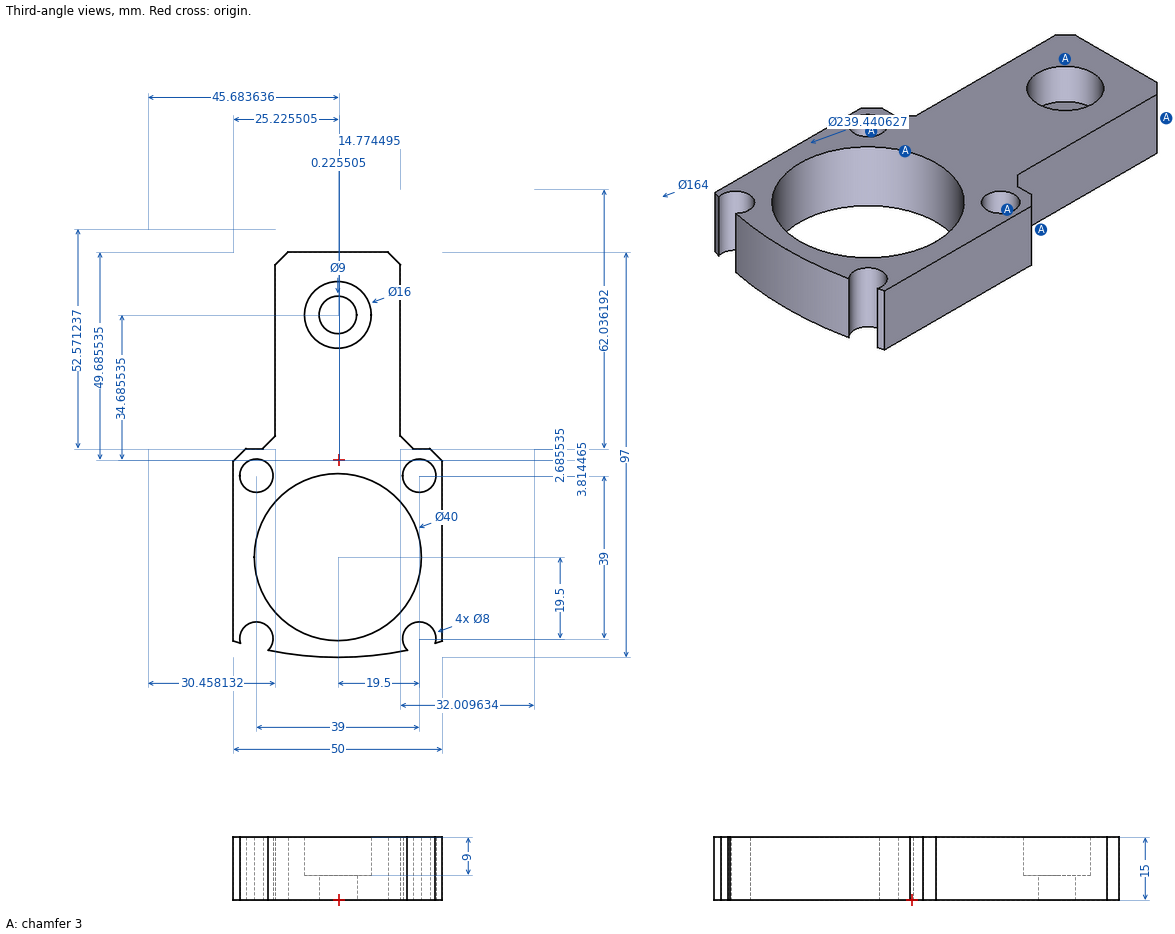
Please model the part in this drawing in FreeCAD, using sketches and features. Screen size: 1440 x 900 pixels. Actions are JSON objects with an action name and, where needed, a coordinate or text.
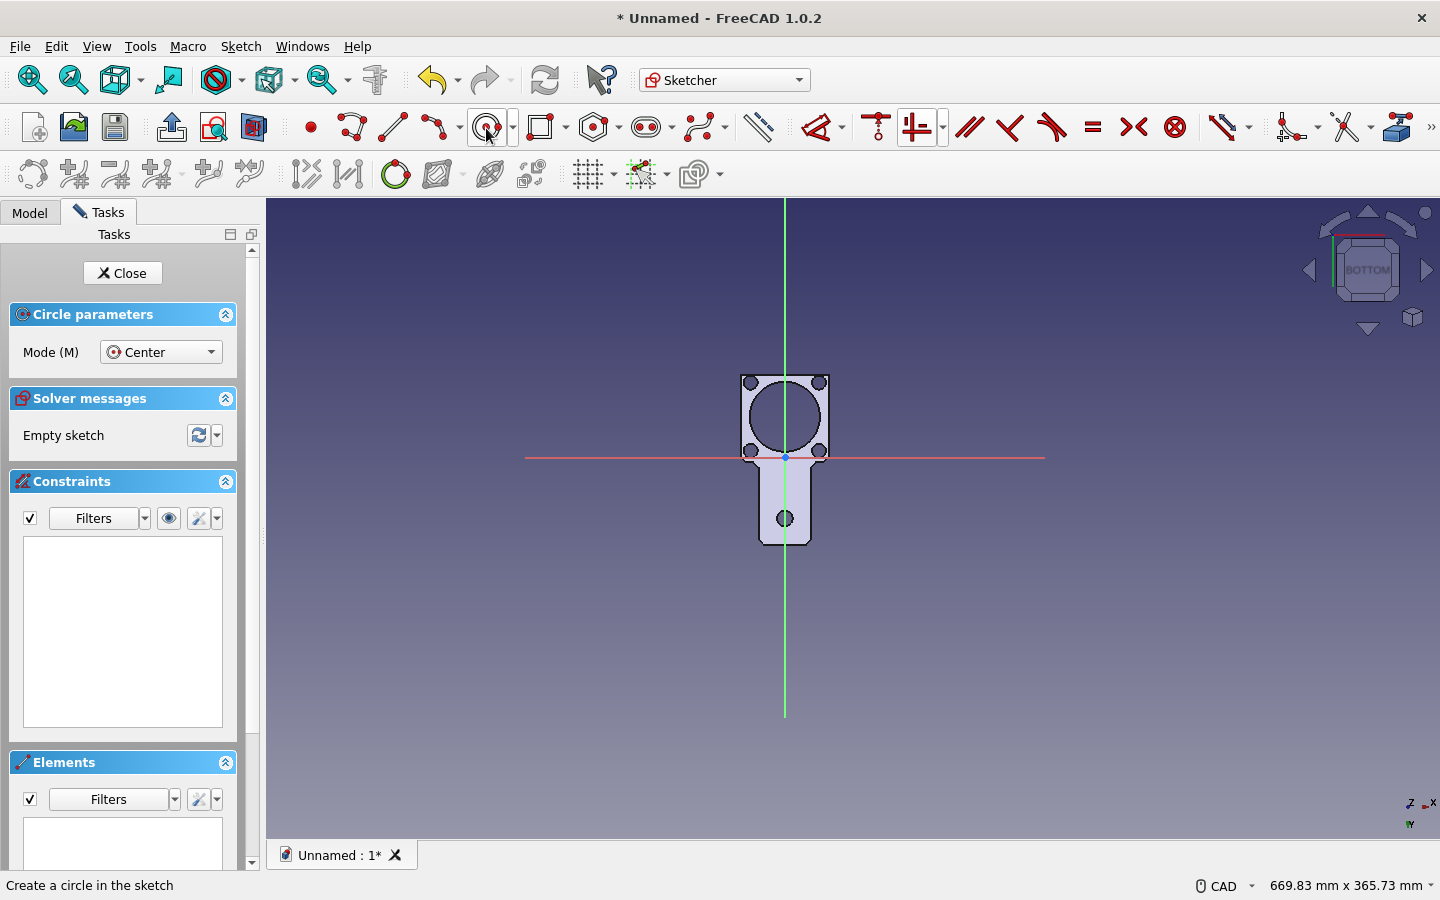
{"action": "scroll", "coordinate": [785, 518], "scroll_direction": "up", "scroll_amount": 19}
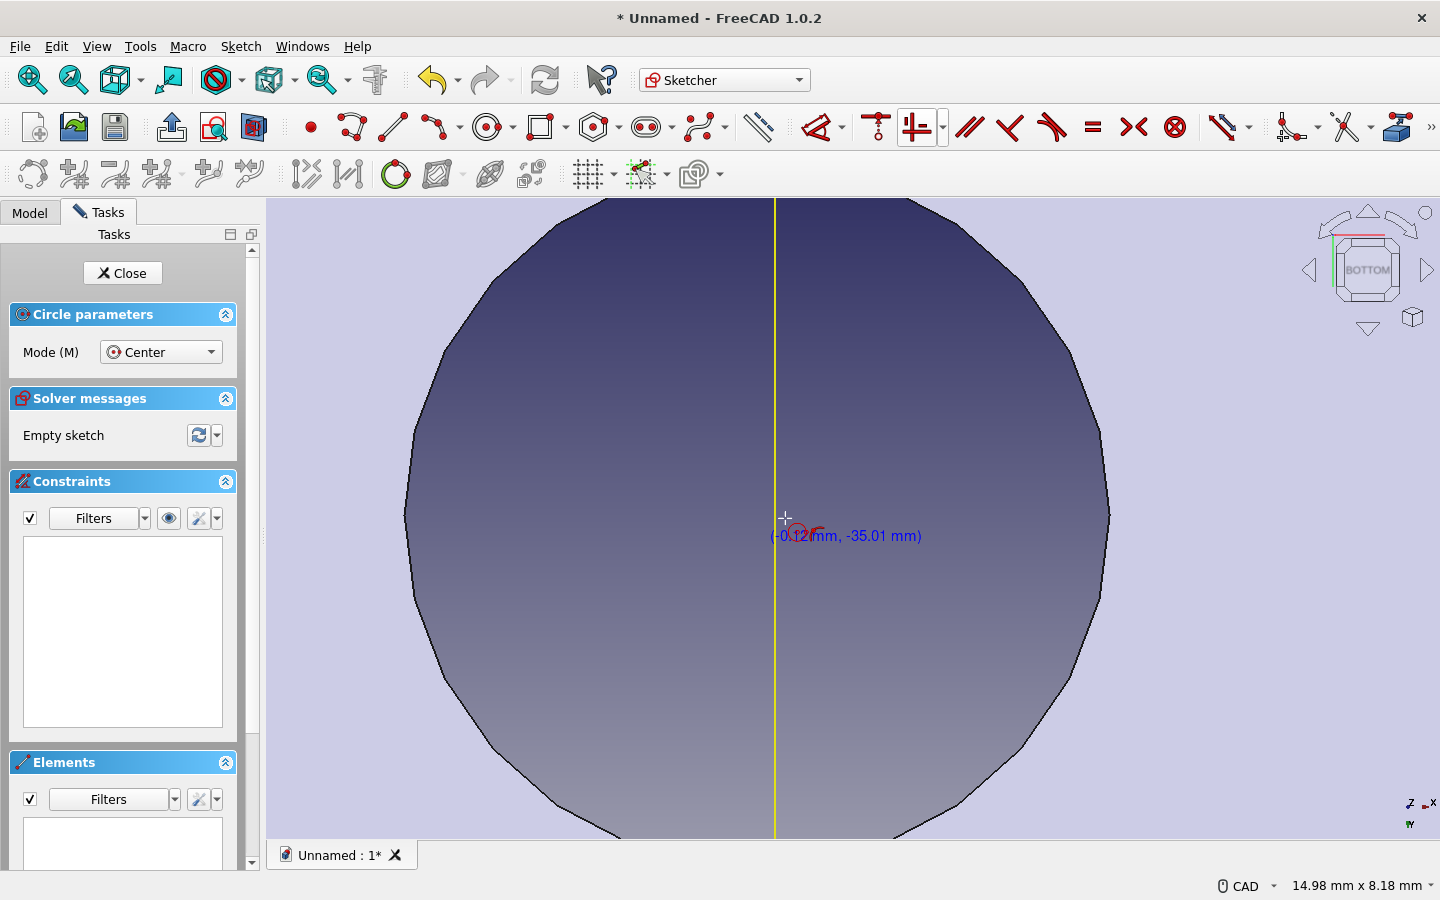
{"action": "left_click", "coordinate": [757, 515]}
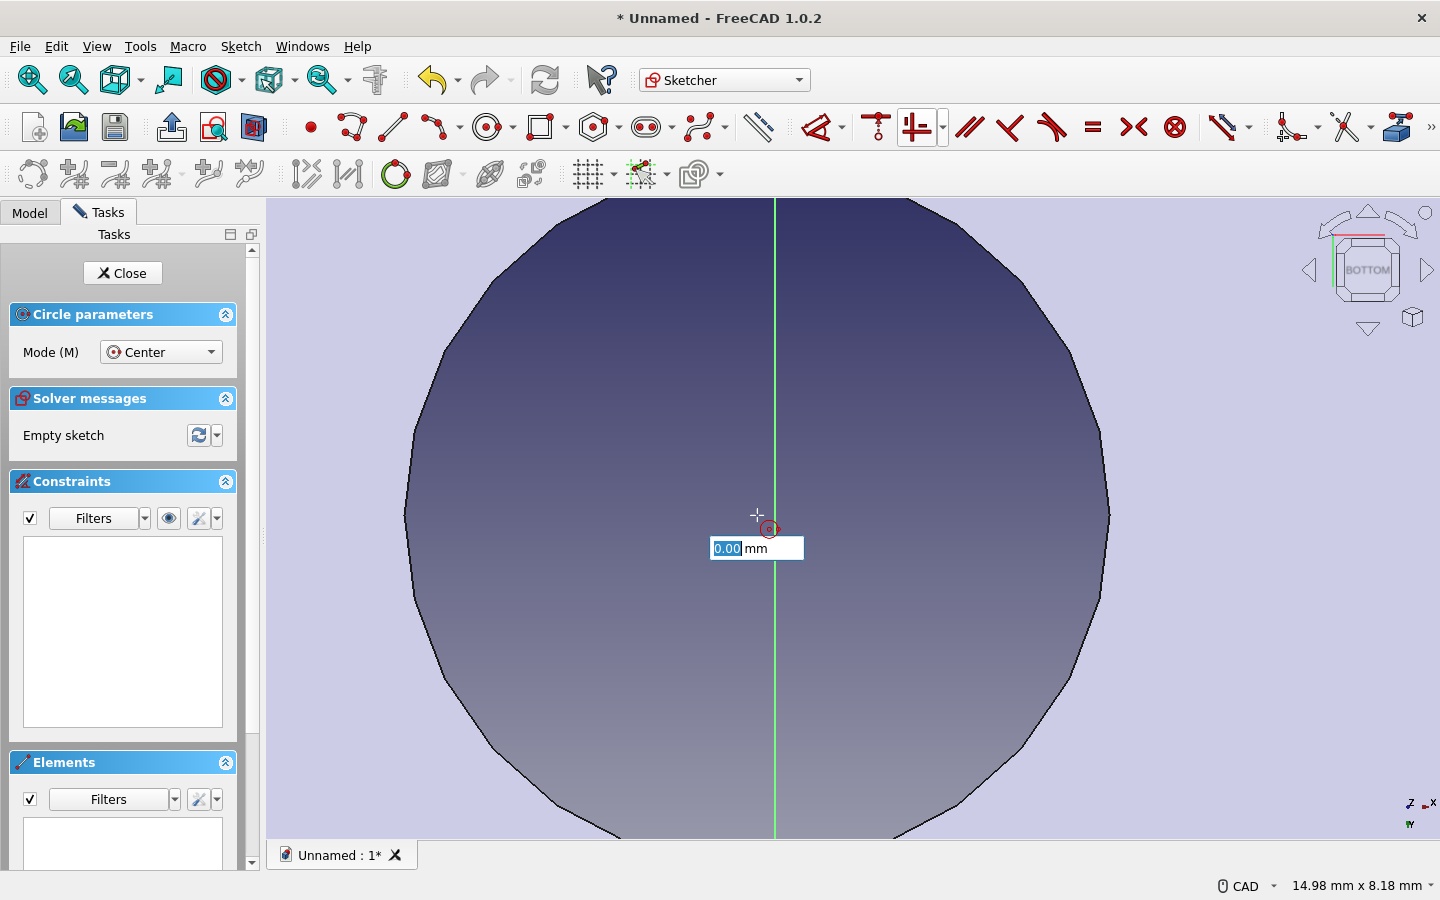
{"action": "scroll", "coordinate": [785, 519], "scroll_direction": "down", "scroll_amount": 18}
{"action": "mouse_move", "coordinate": [966, 338]}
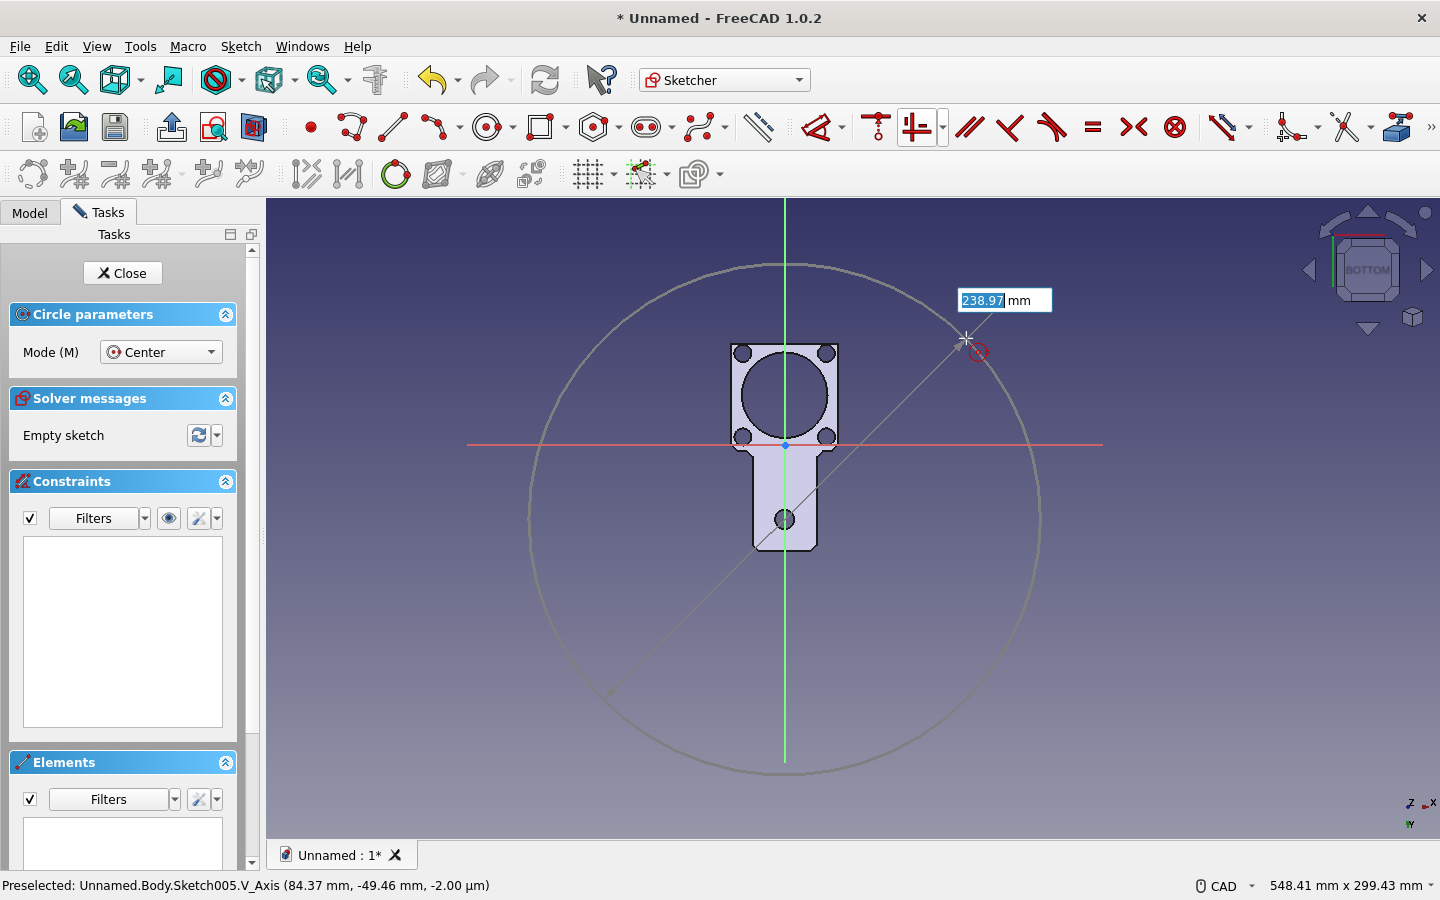
{"action": "type", "text": "239.440627"}
{"action": "key", "text": "Return"}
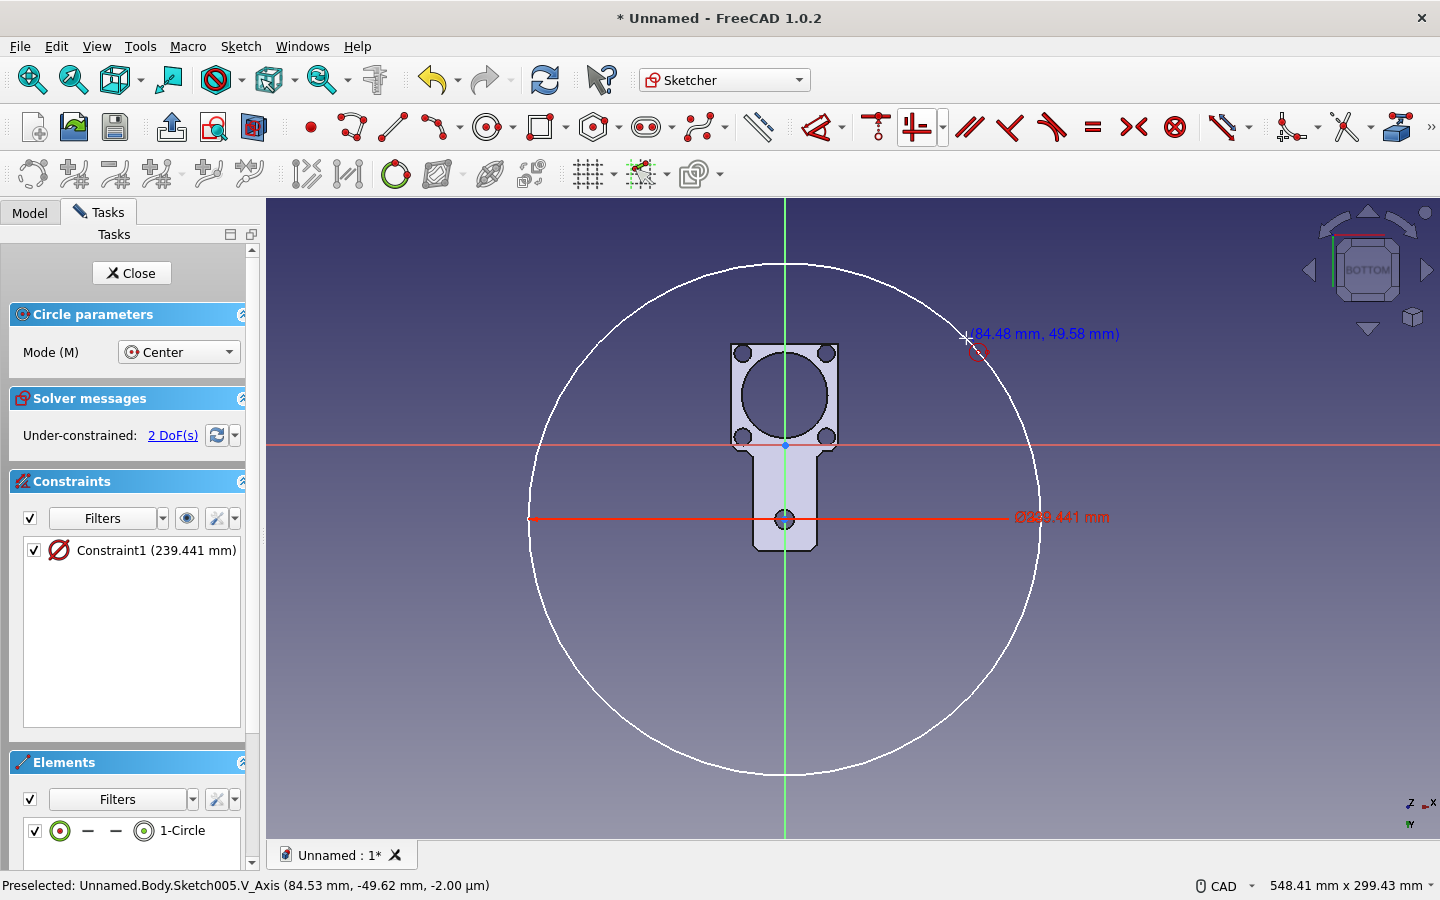
{"action": "scroll", "coordinate": [785, 519], "scroll_direction": "up", "scroll_amount": 18}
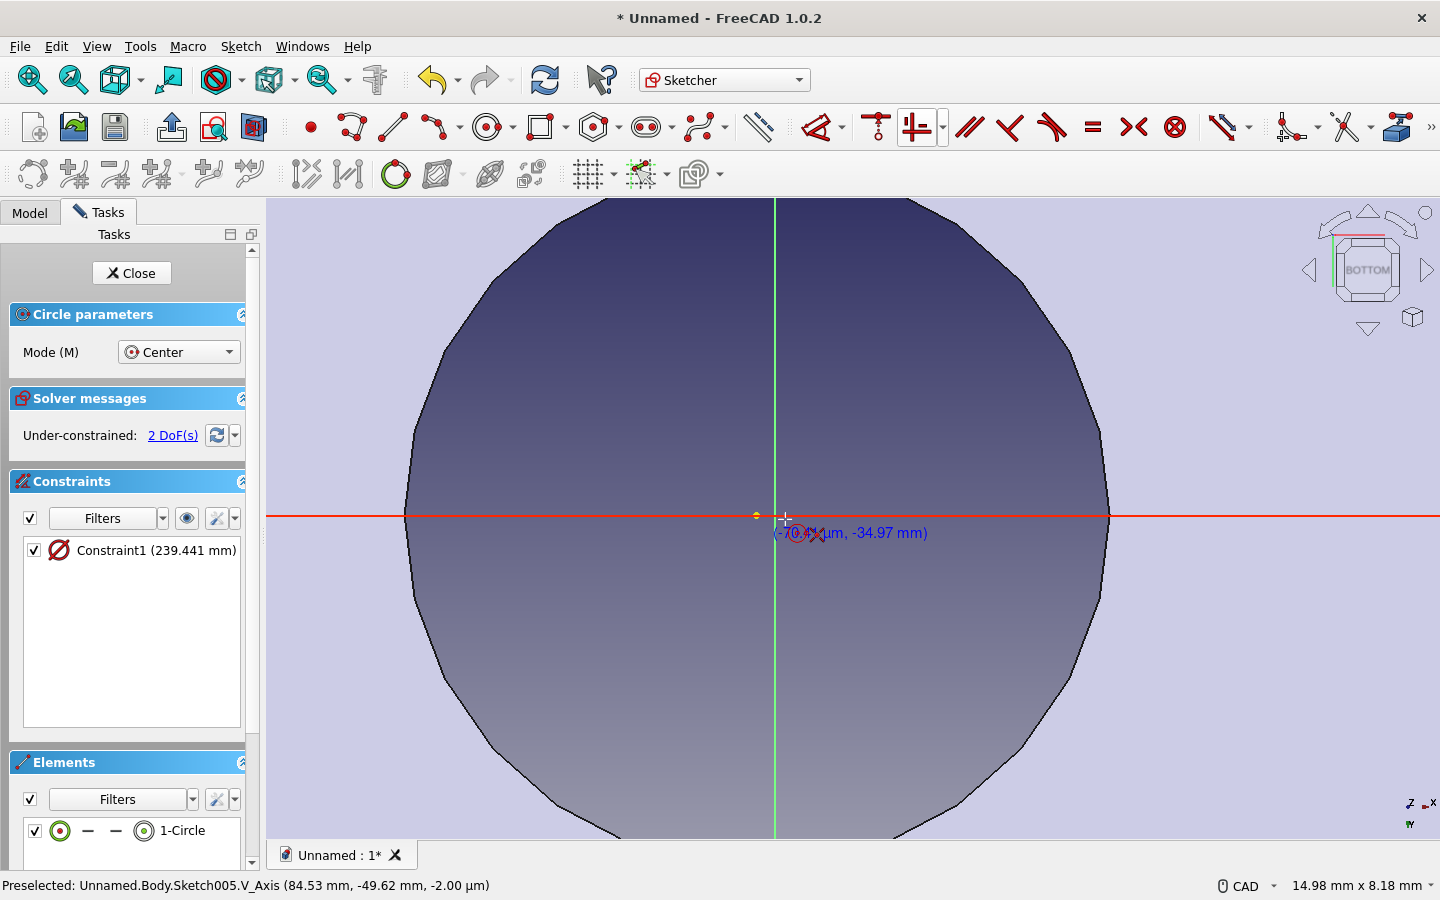
{"action": "left_click", "coordinate": [757, 516]}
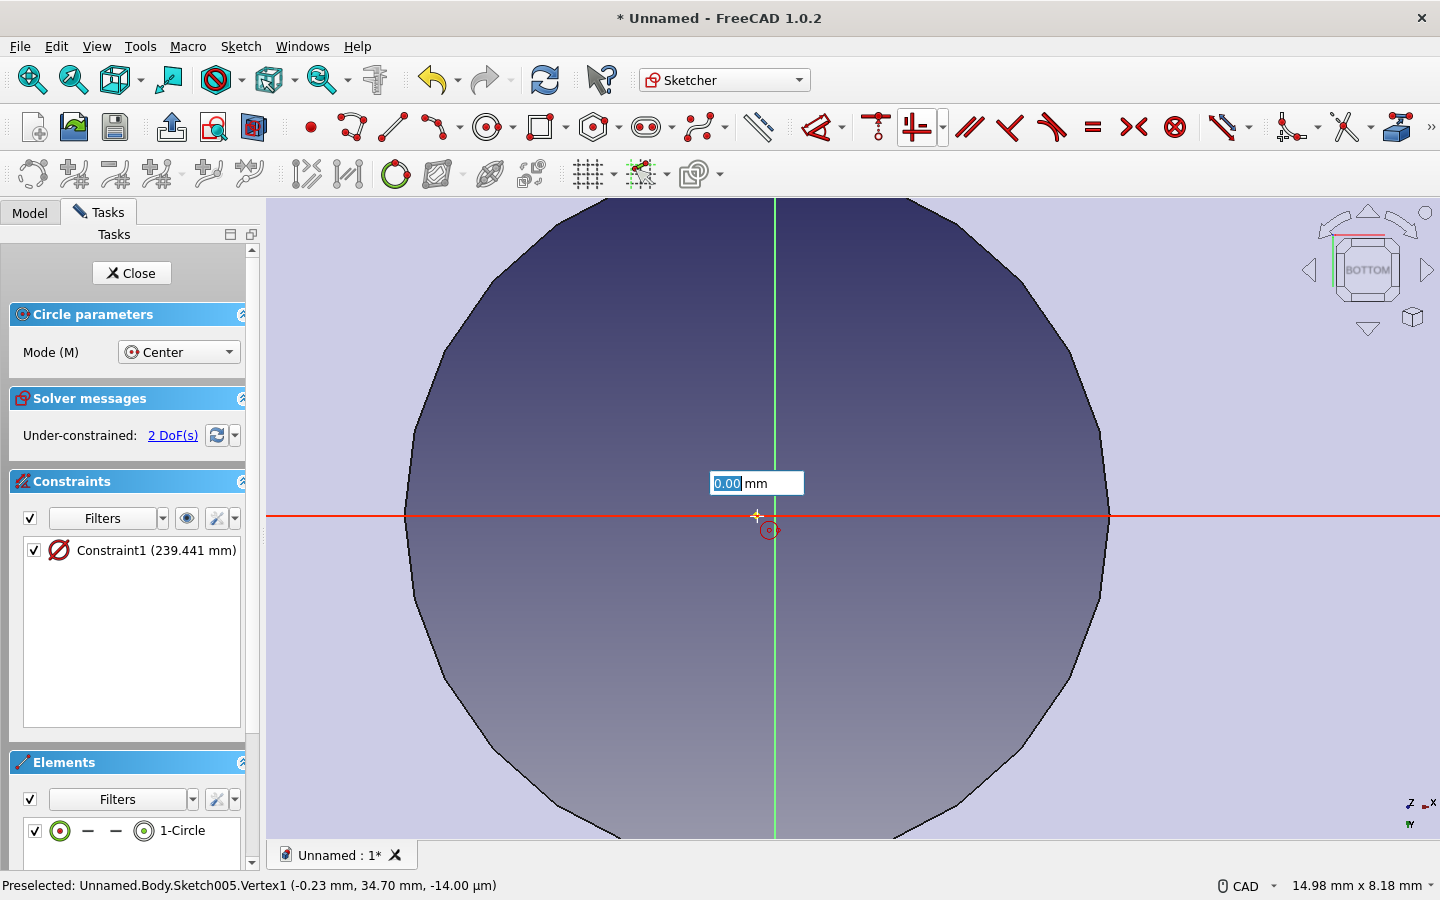
{"action": "scroll", "coordinate": [785, 519], "scroll_direction": "down", "scroll_amount": 18}
{"action": "mouse_move", "coordinate": [909, 395]}